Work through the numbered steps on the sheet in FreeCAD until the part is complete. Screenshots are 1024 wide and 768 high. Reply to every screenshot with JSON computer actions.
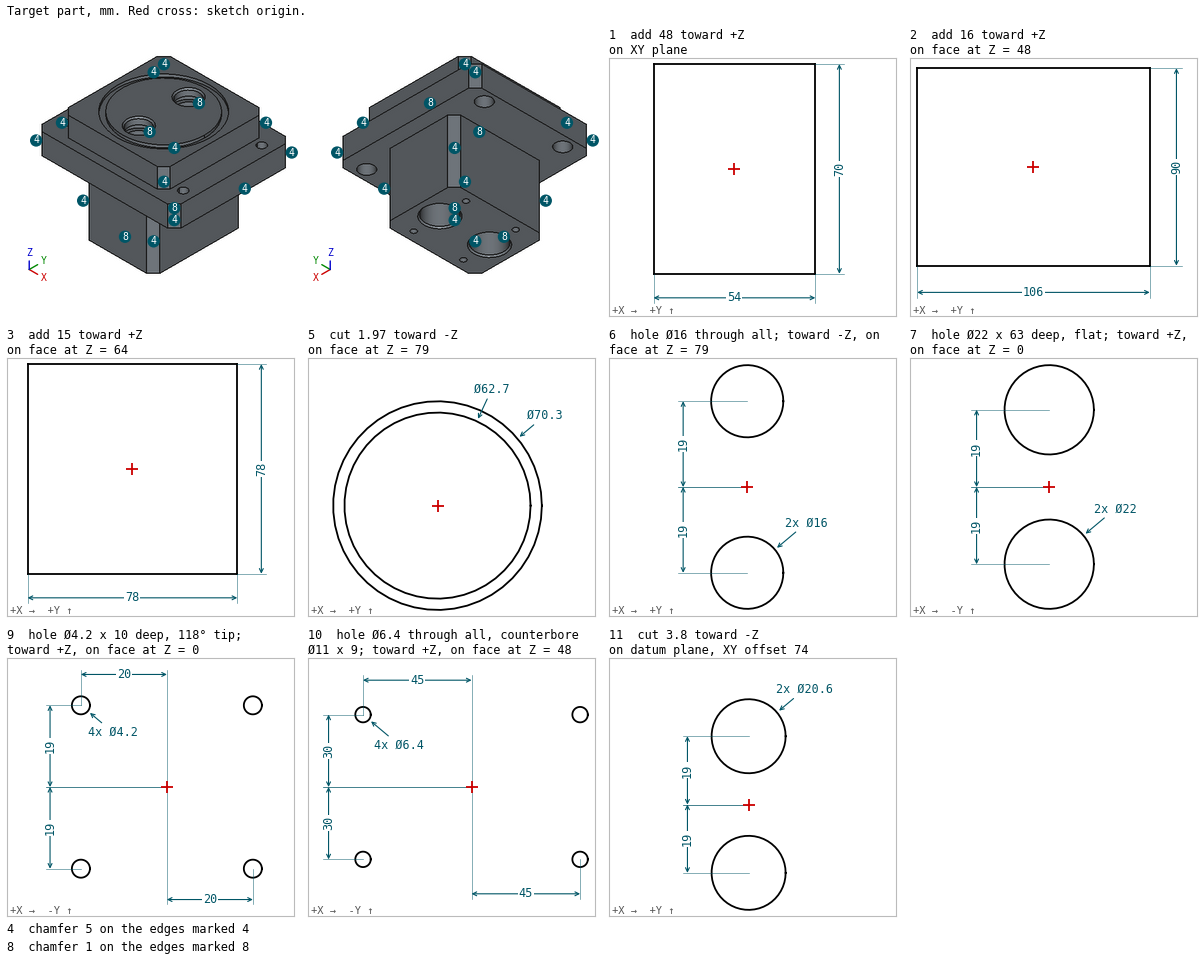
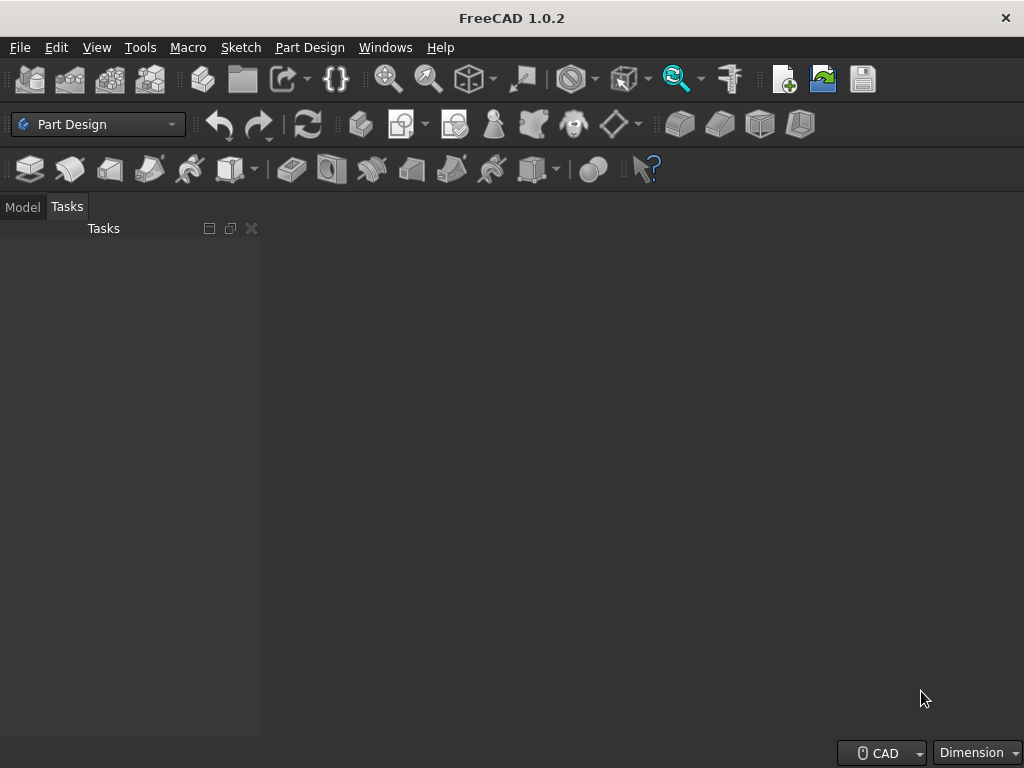
{"action": "left_click", "coordinate": [784, 80]}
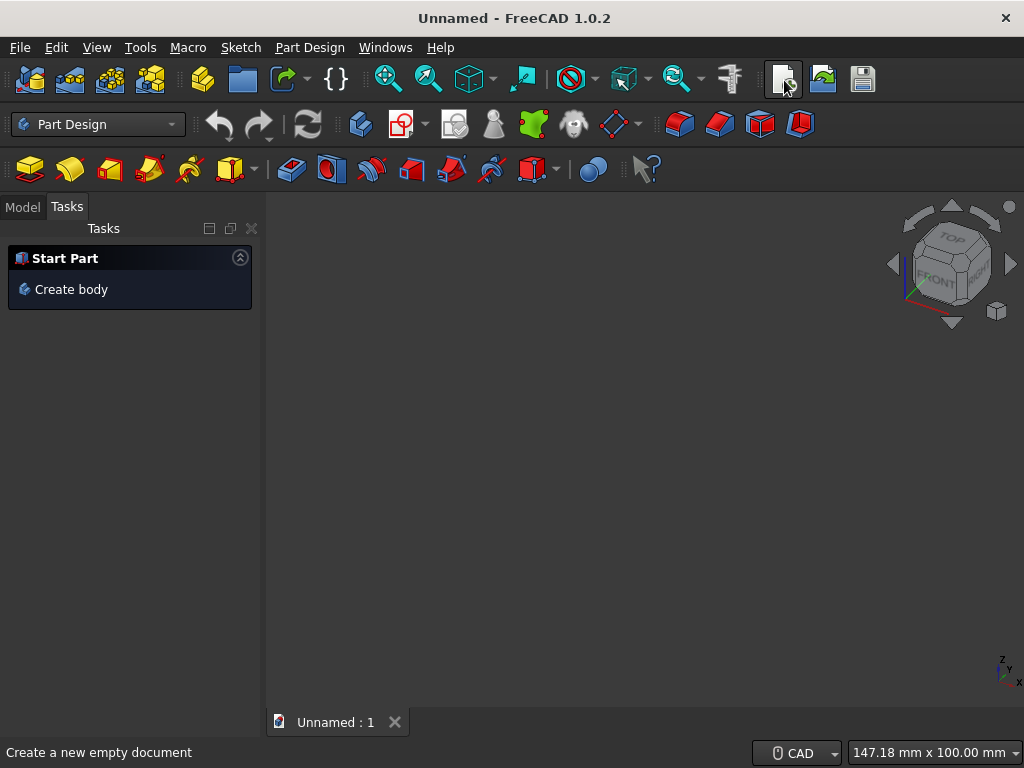
{"action": "left_click", "coordinate": [402, 124]}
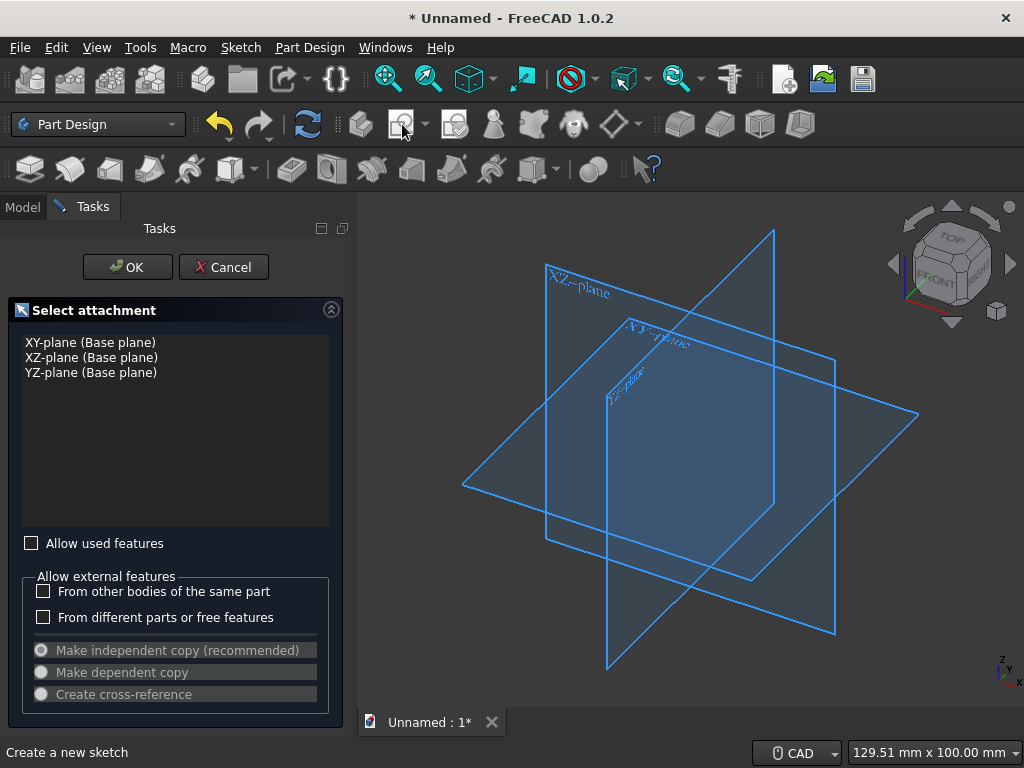
{"action": "left_click", "coordinate": [82, 342]}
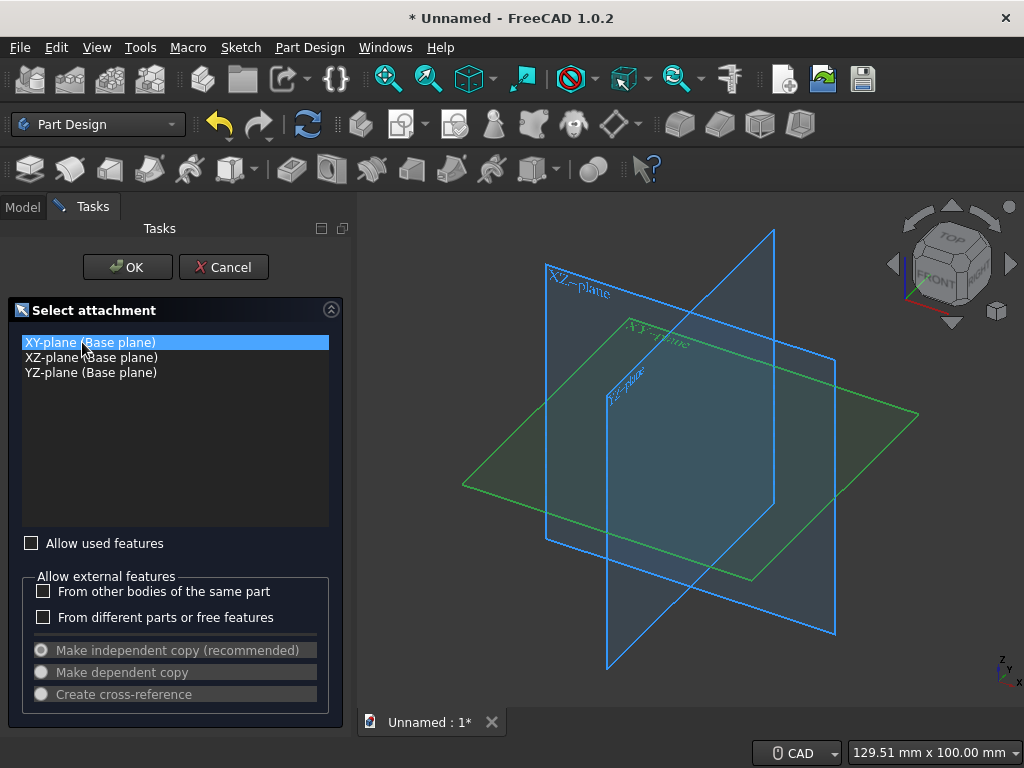
{"action": "left_click", "coordinate": [128, 267]}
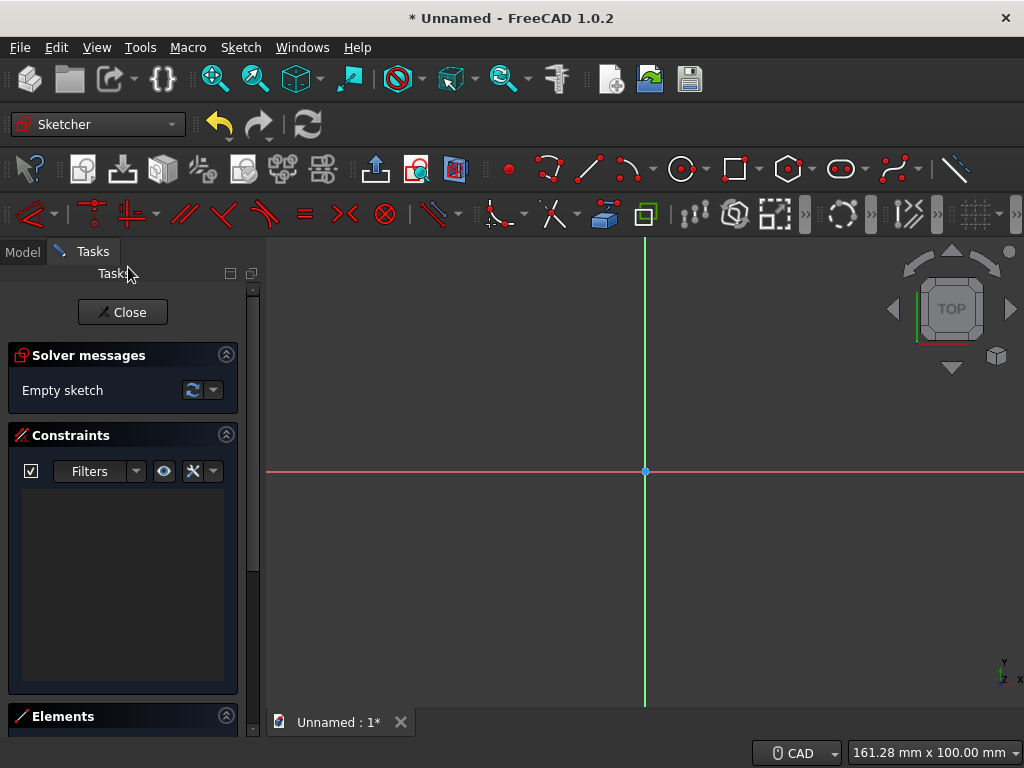
{"action": "key", "text": "g v"}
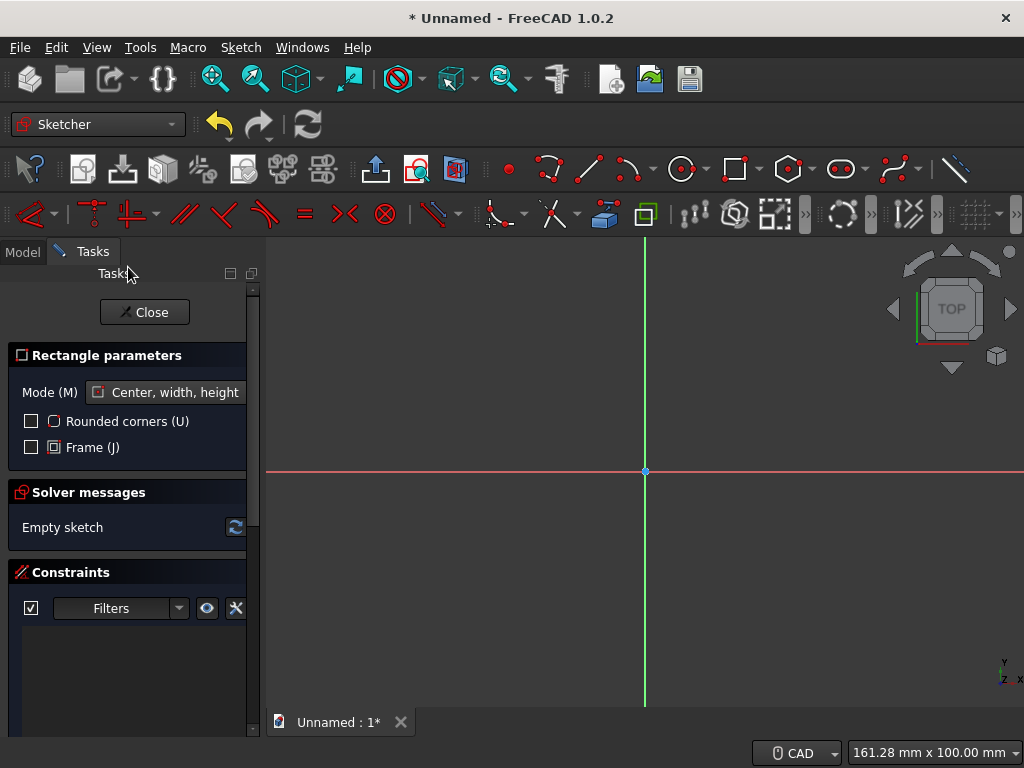
{"action": "left_click", "coordinate": [645, 472]}
{"action": "mouse_move", "coordinate": [772, 308]}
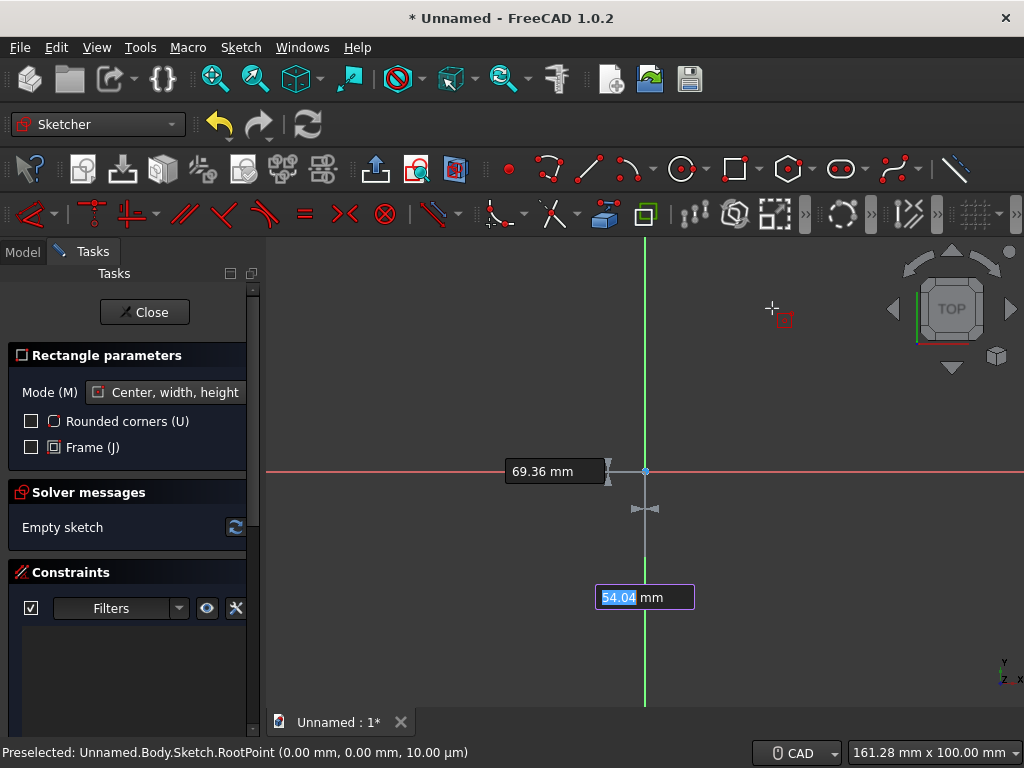
{"action": "type", "text": "54"}
{"action": "key", "text": "Tab"}
{"action": "type", "text": "70"}
{"action": "key", "text": "Return"}
{"action": "key", "text": "Escape"}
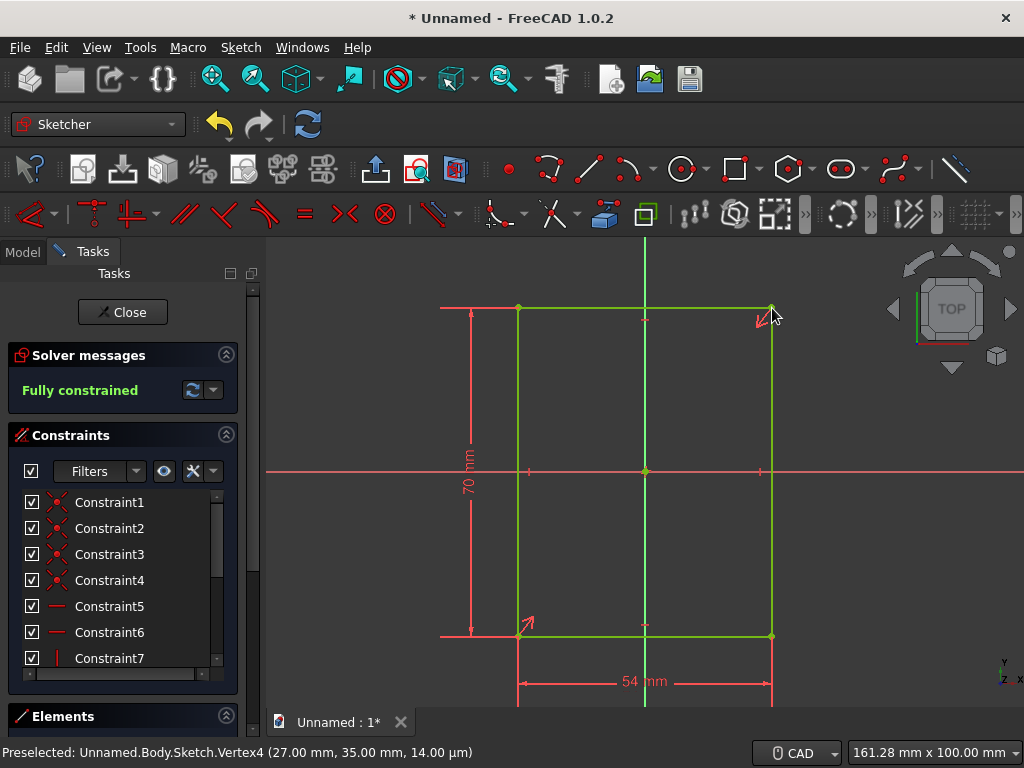
{"action": "left_click", "coordinate": [123, 312]}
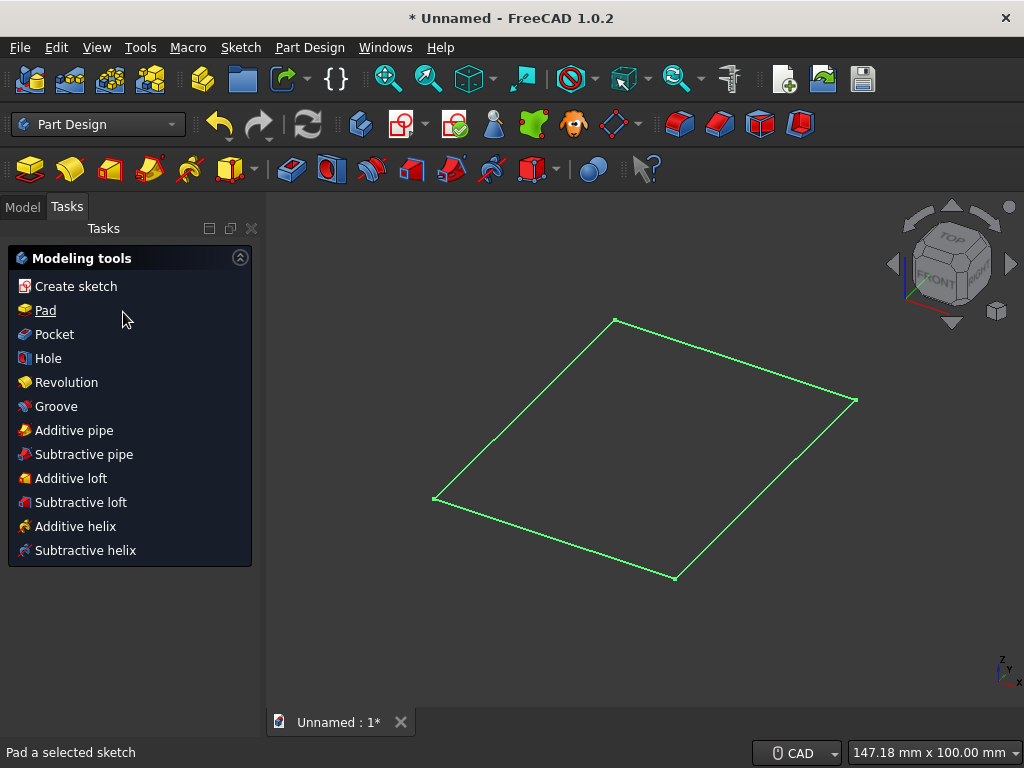
{"action": "left_click", "coordinate": [30, 170]}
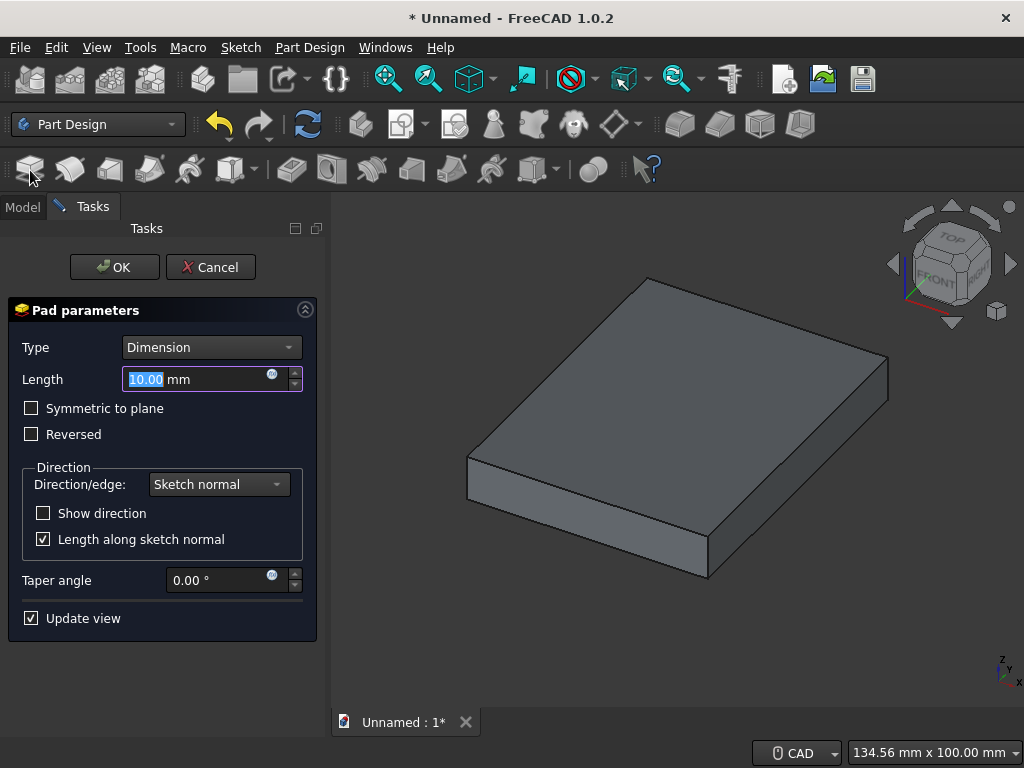
{"action": "type", "text": "48"}
{"action": "key", "text": "Tab"}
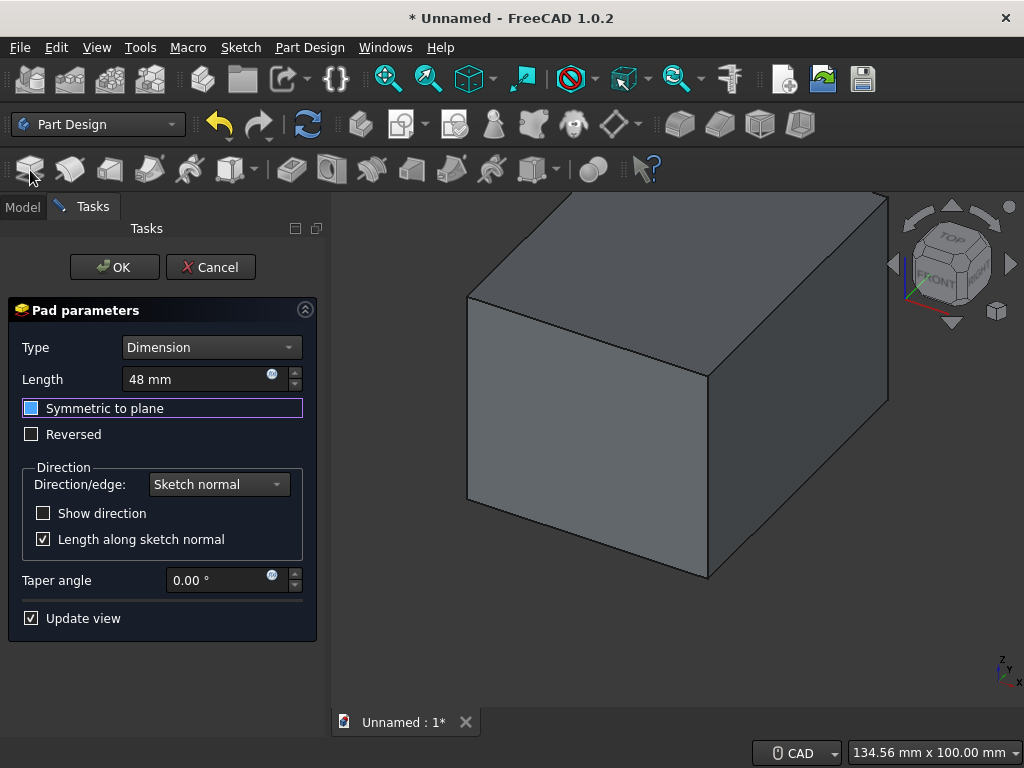
{"action": "left_click", "coordinate": [115, 267]}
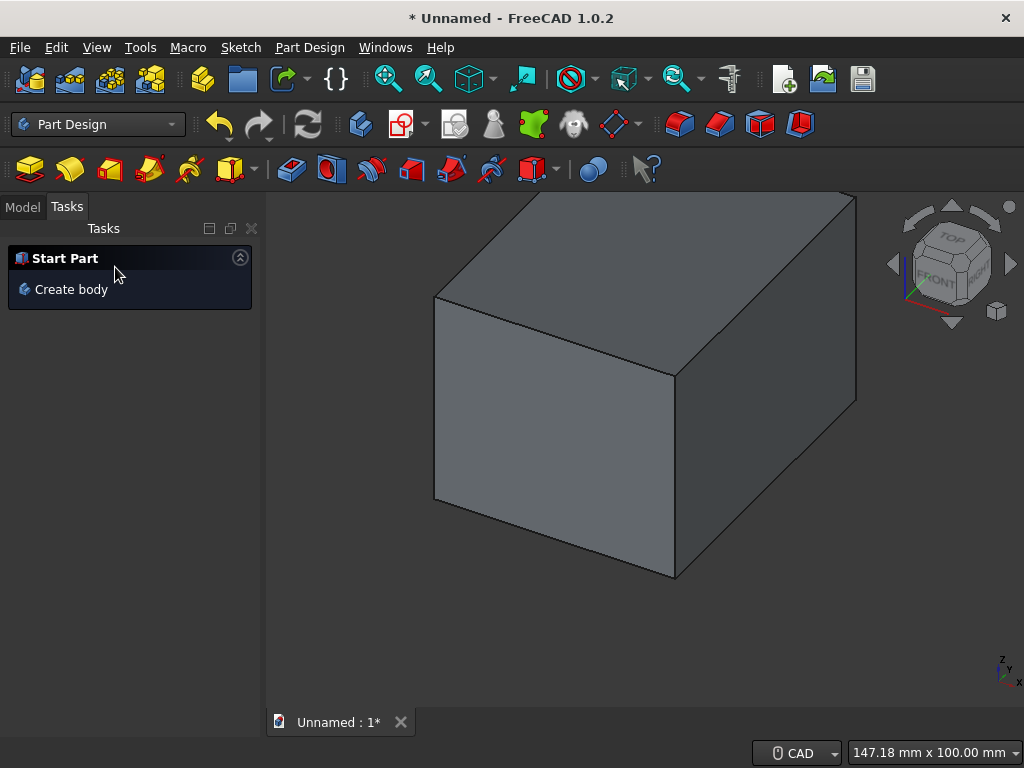
{"action": "left_click", "coordinate": [390, 80]}